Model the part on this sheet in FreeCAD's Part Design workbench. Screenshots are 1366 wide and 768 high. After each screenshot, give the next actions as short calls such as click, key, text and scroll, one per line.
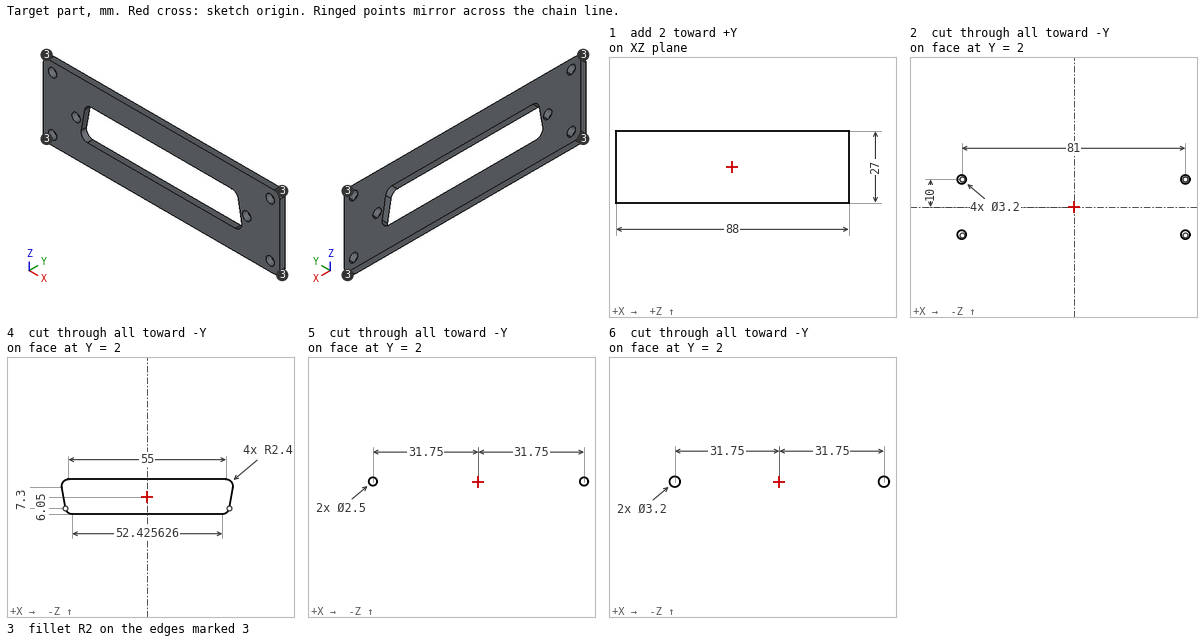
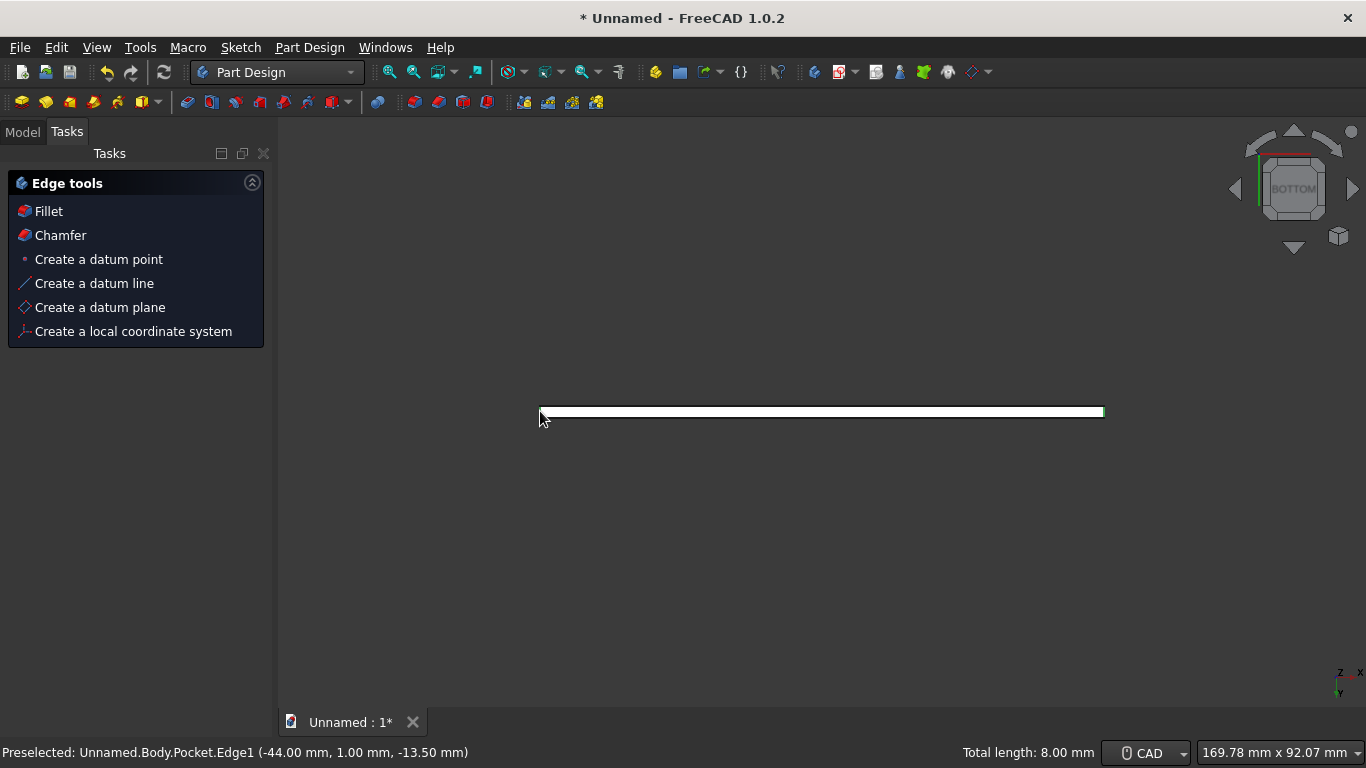
click(416, 102)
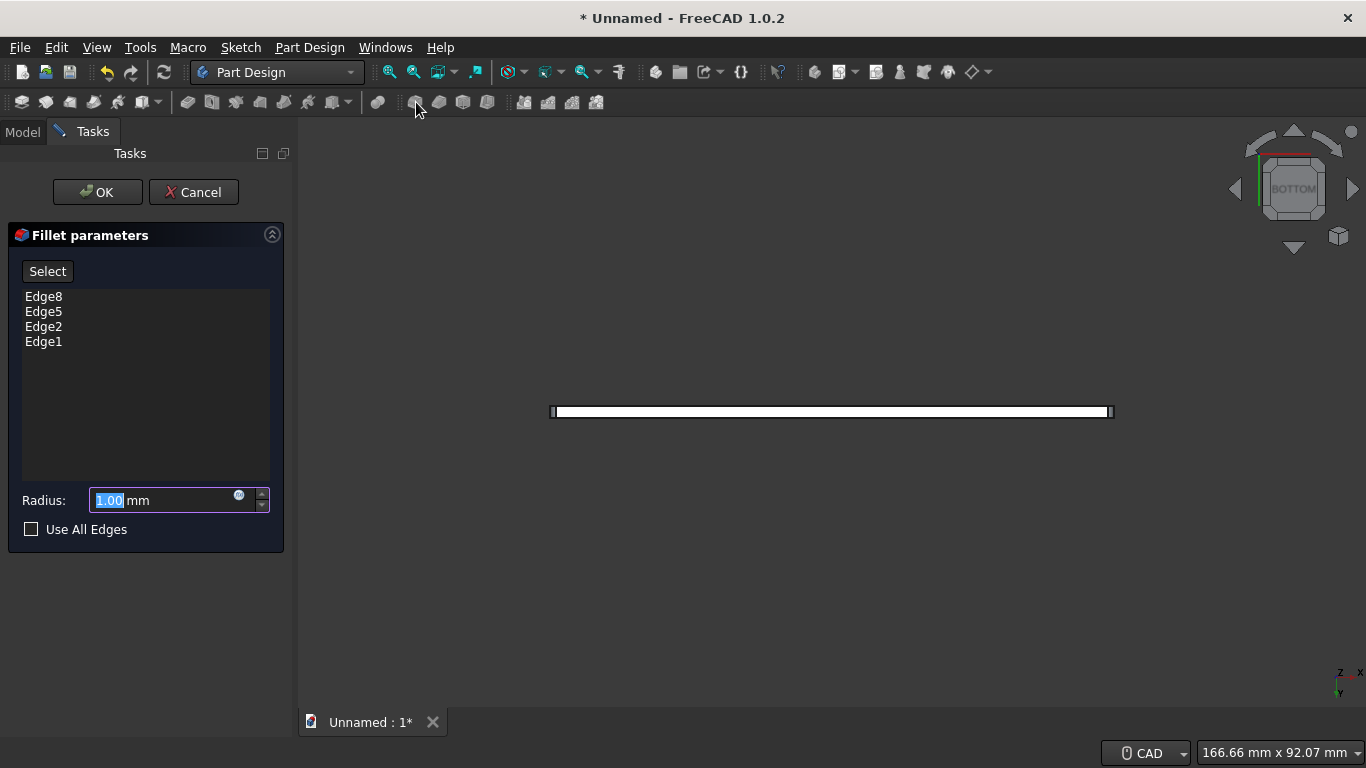
text(2)
key(Tab)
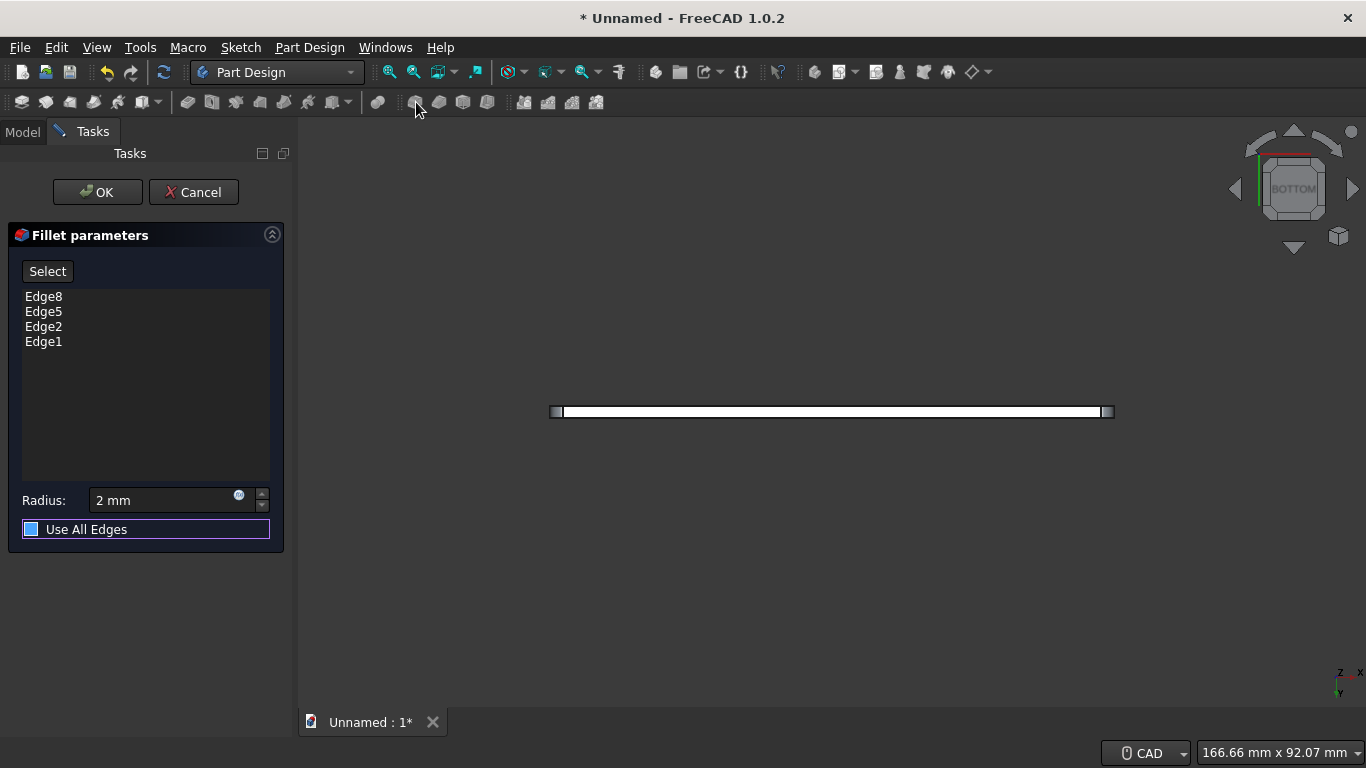
click(98, 192)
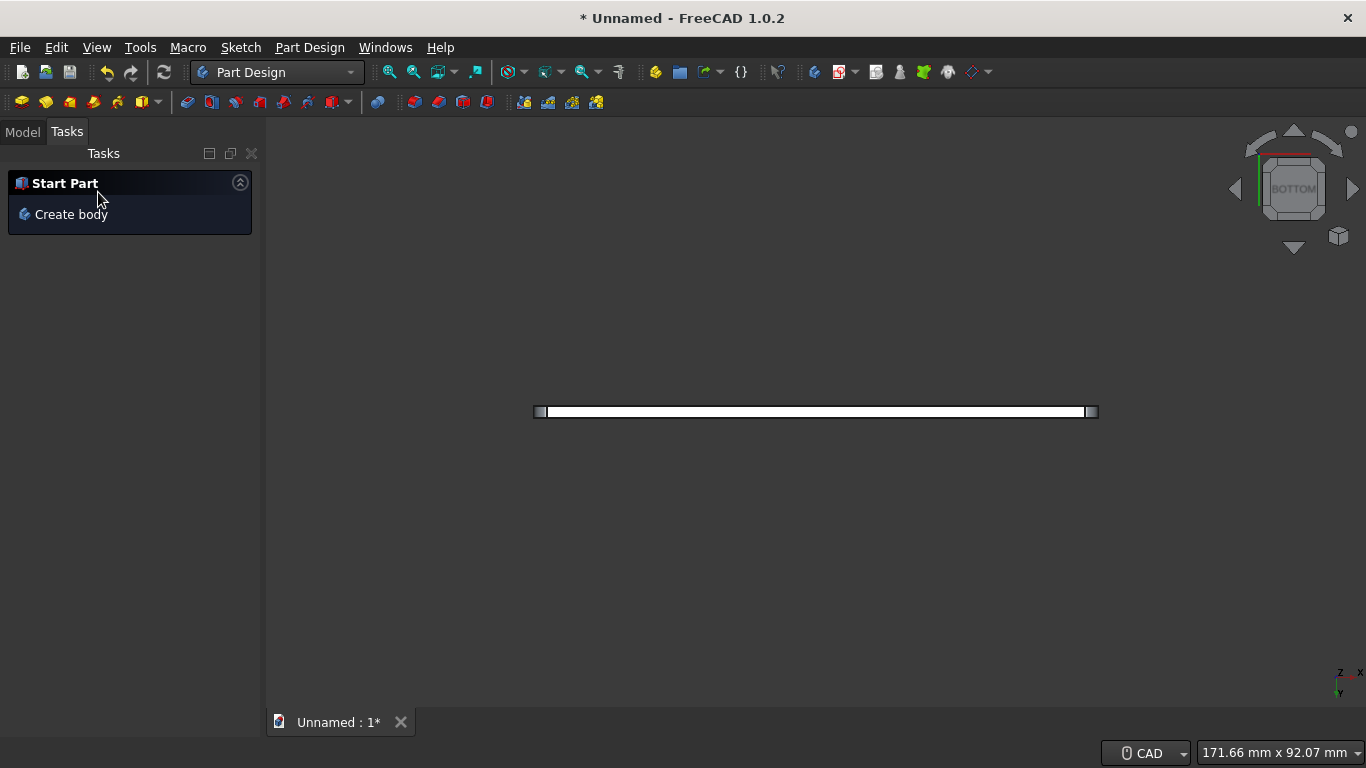
key(4)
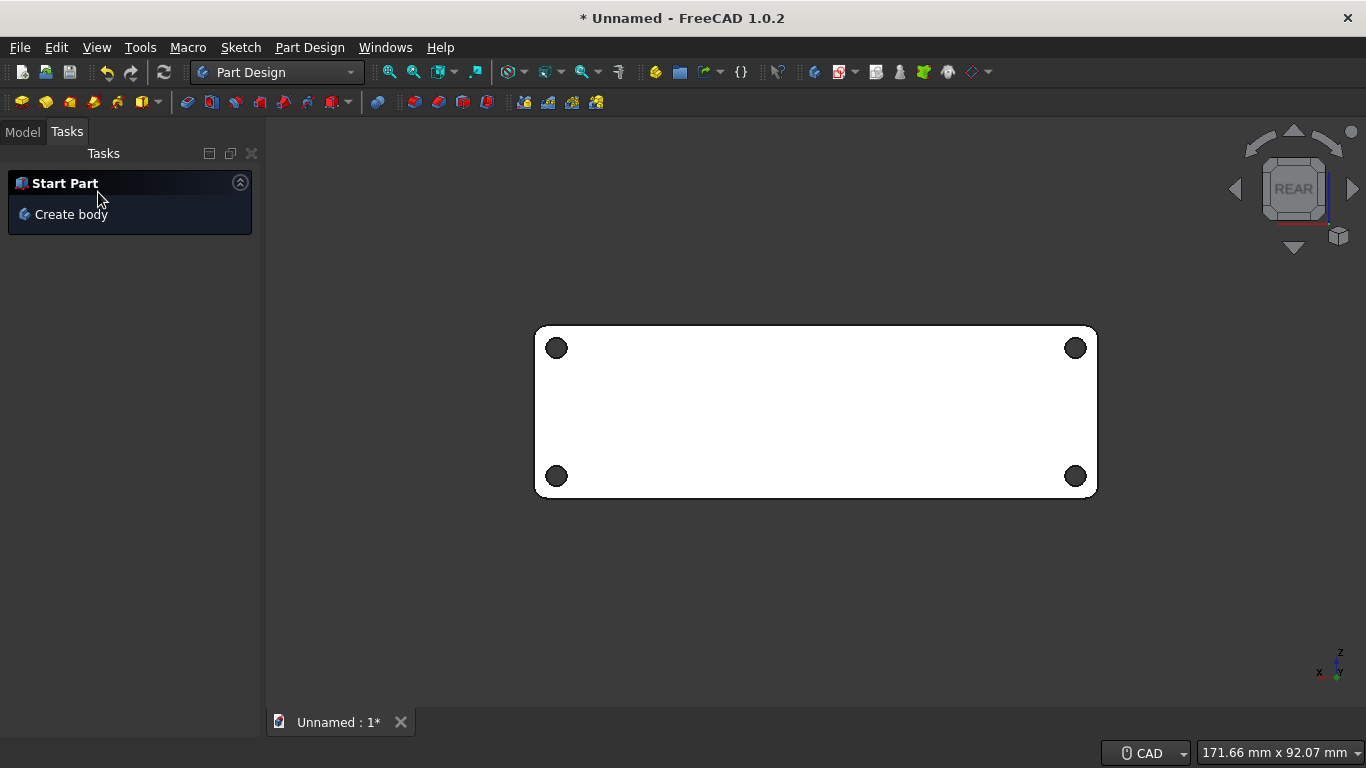
click(655, 411)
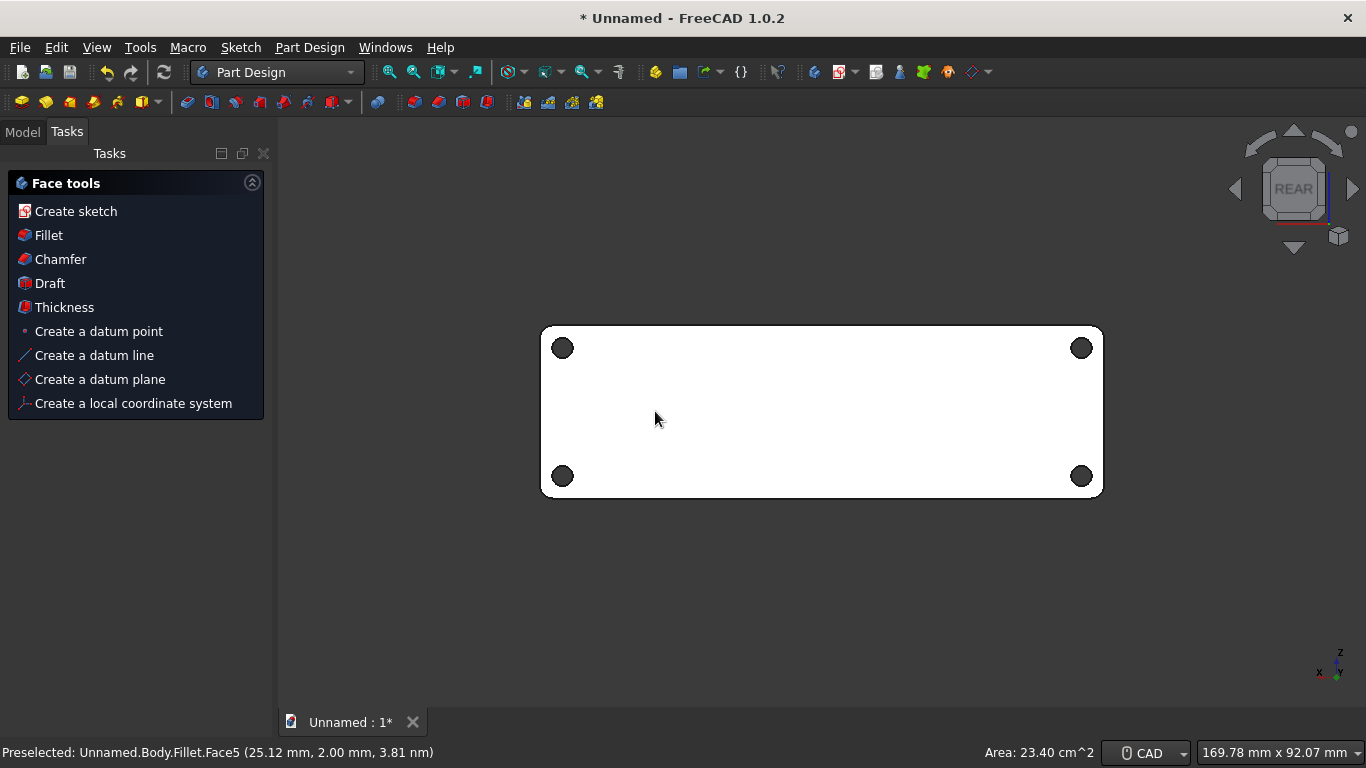
click(840, 72)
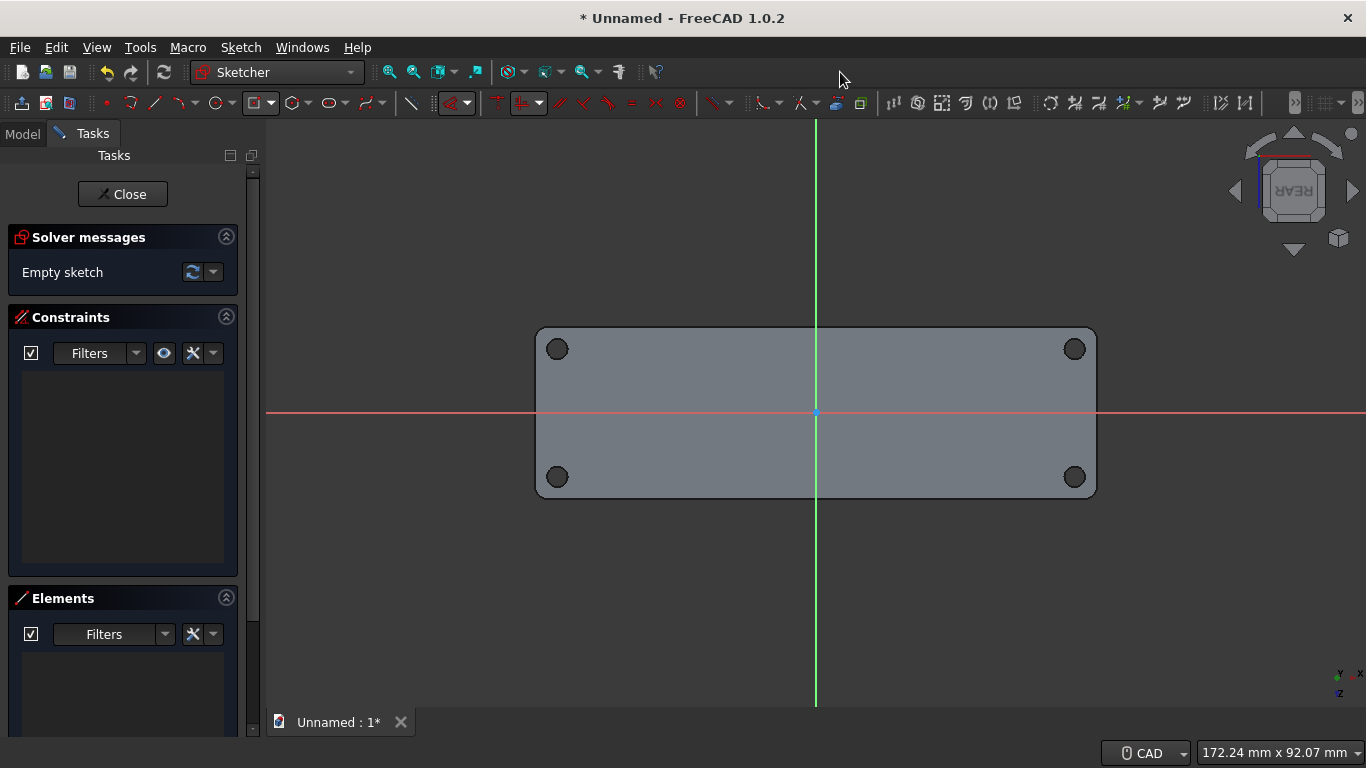
scroll(899, 413, up, 3)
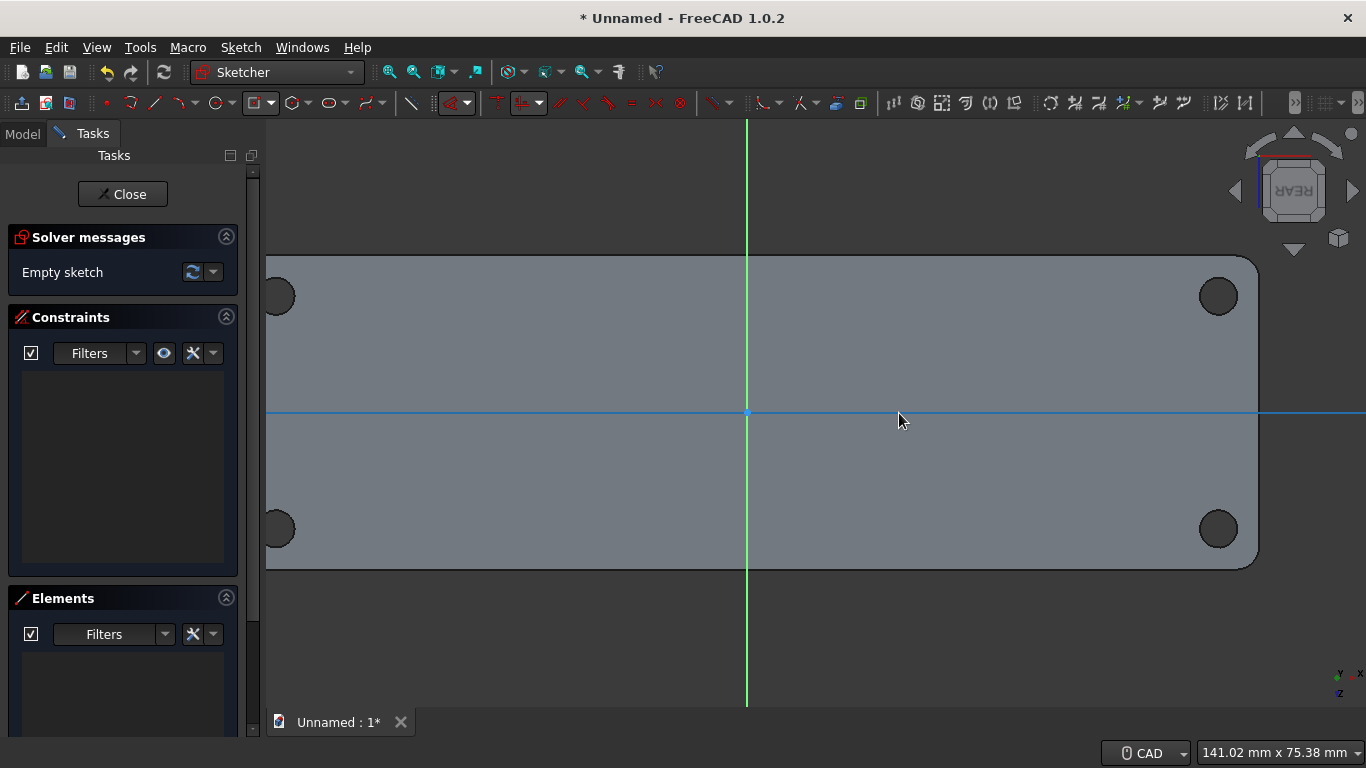
click(156, 104)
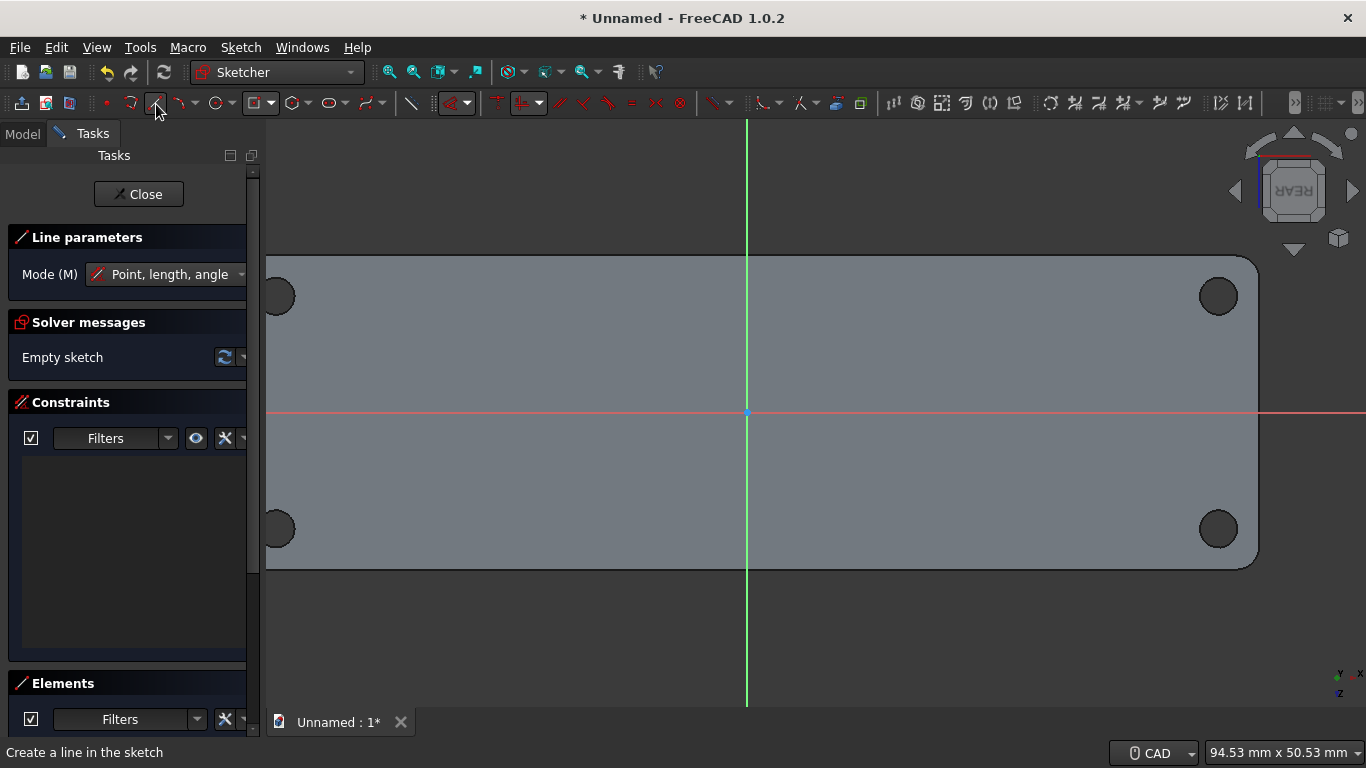
click(400, 375)
click(415, 460)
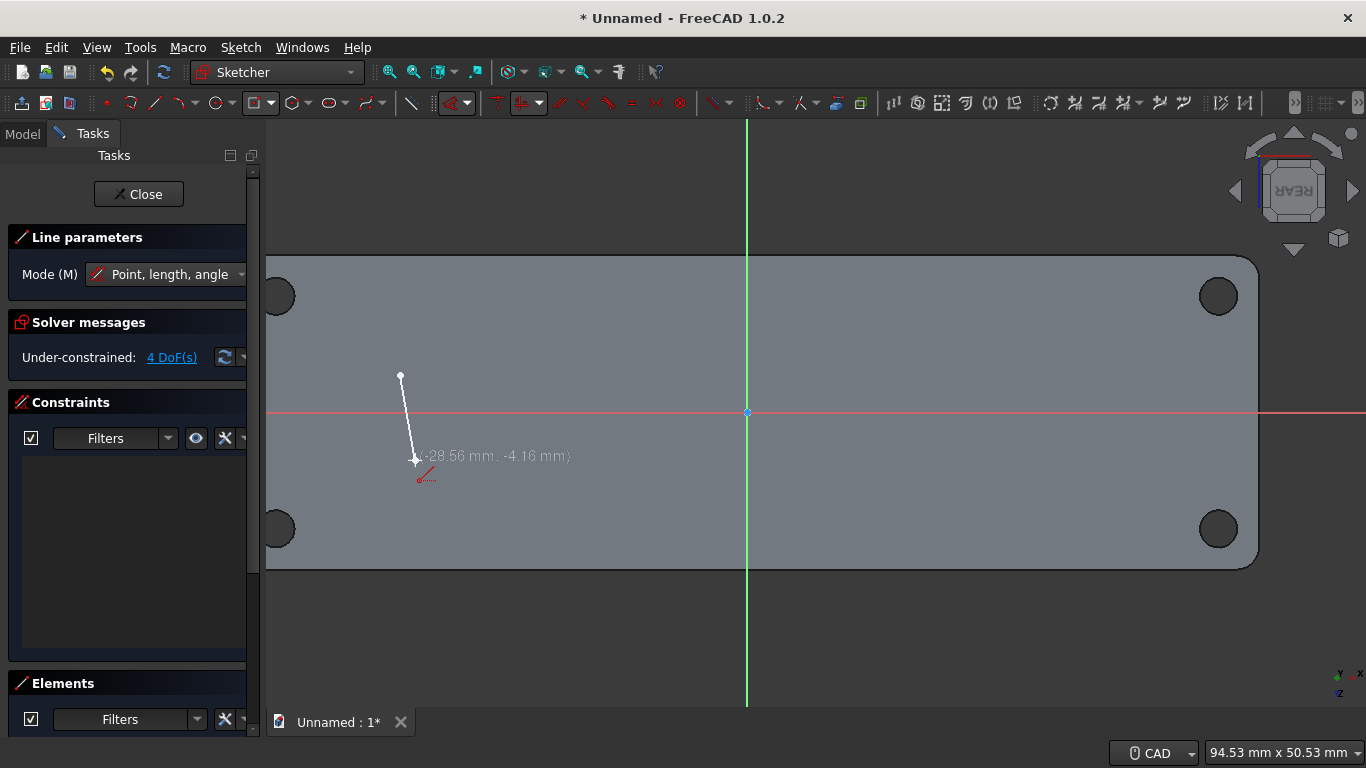
click(442, 483)
click(1052, 483)